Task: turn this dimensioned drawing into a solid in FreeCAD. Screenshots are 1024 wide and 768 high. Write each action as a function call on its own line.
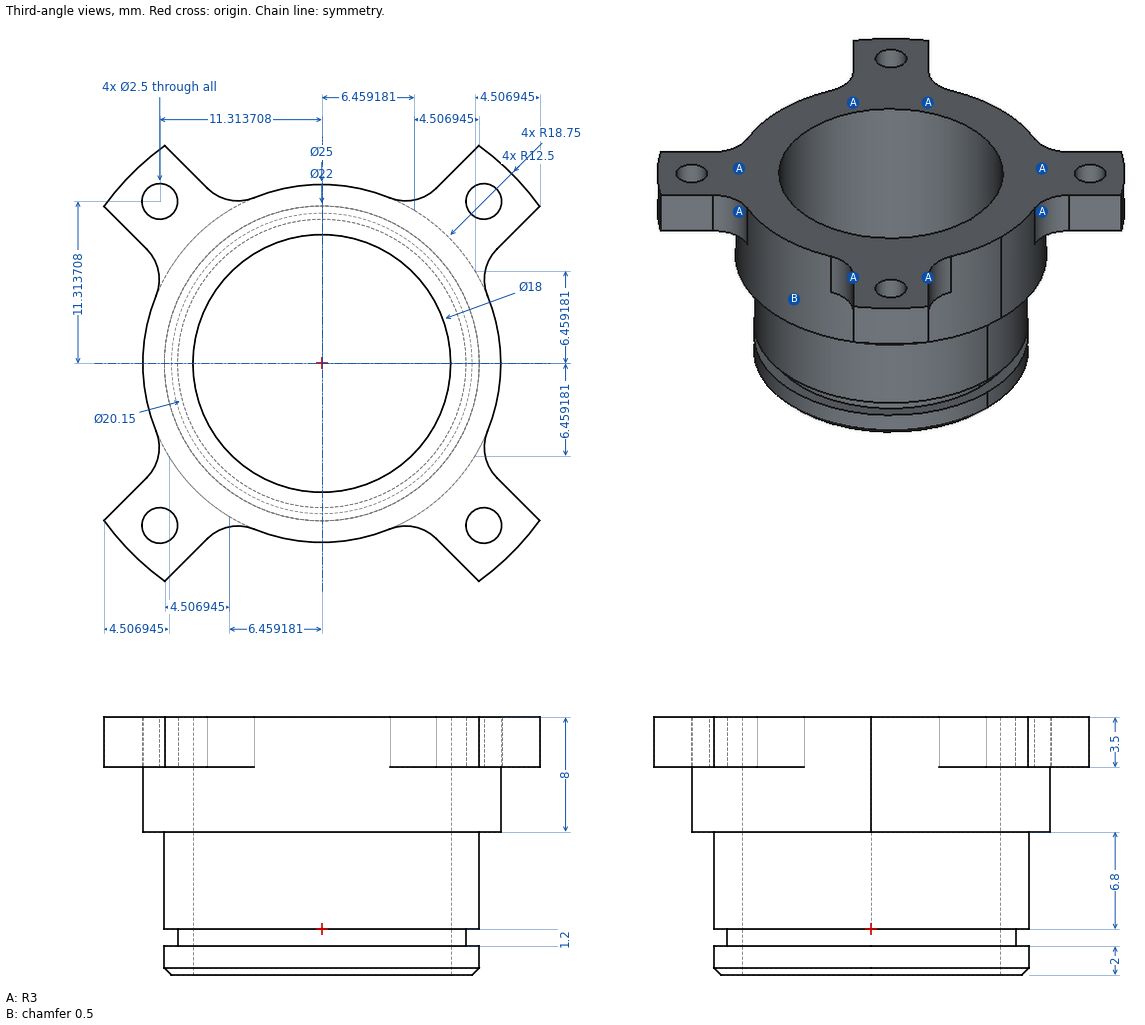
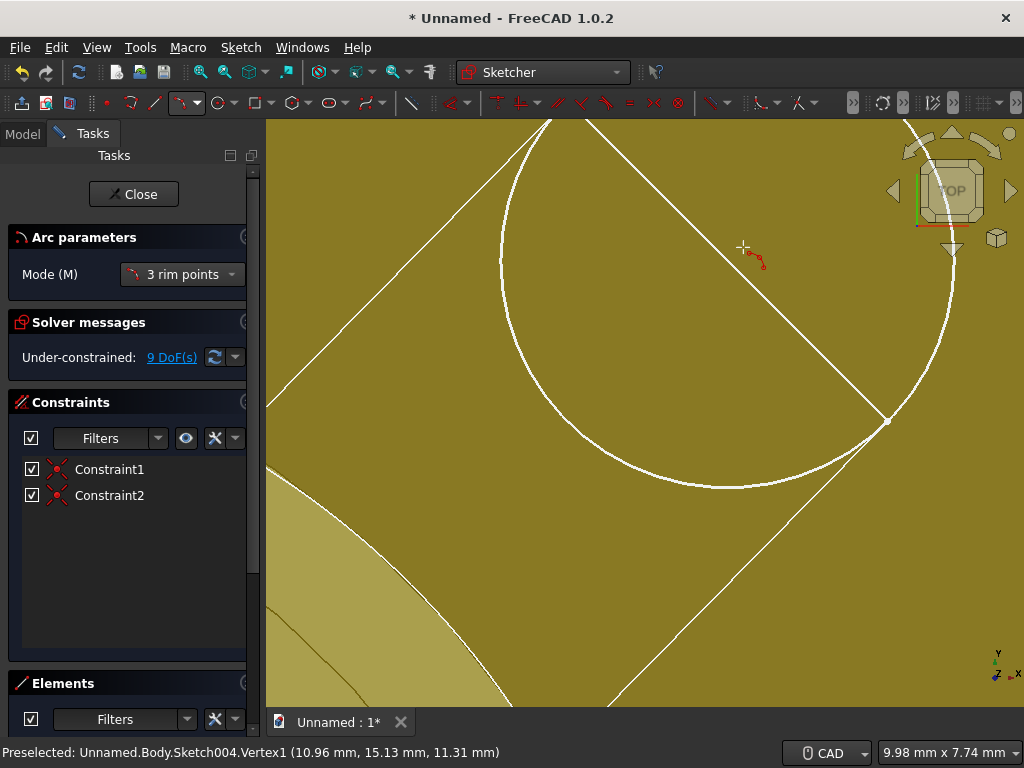
click(742, 243)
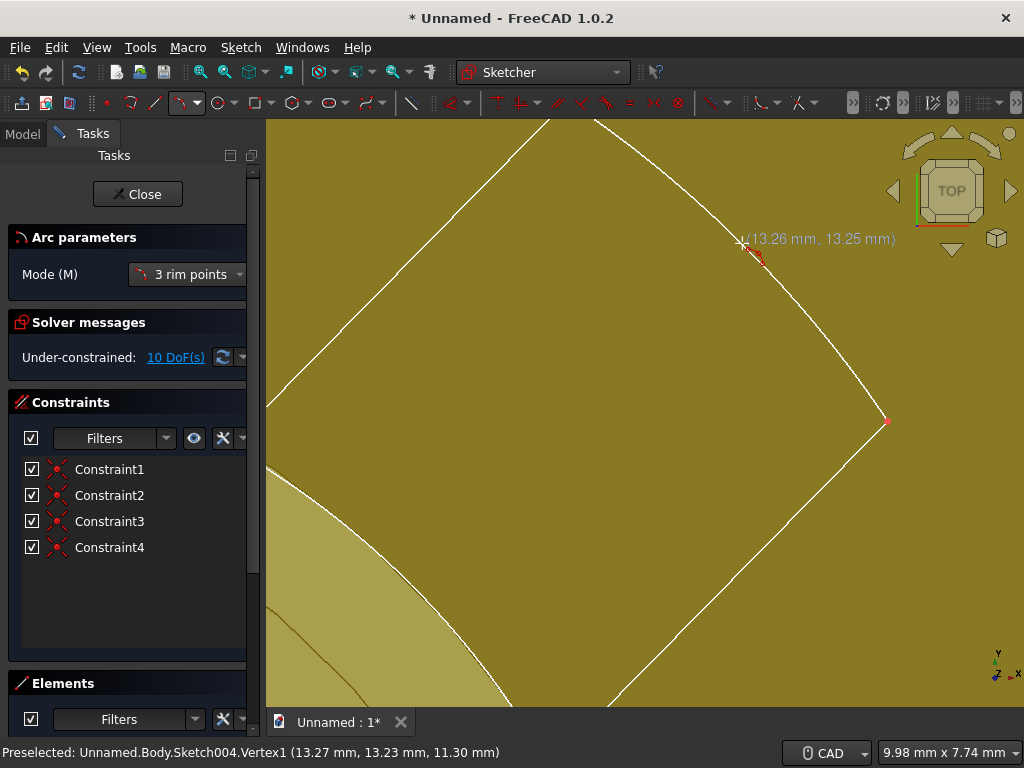
click(156, 104)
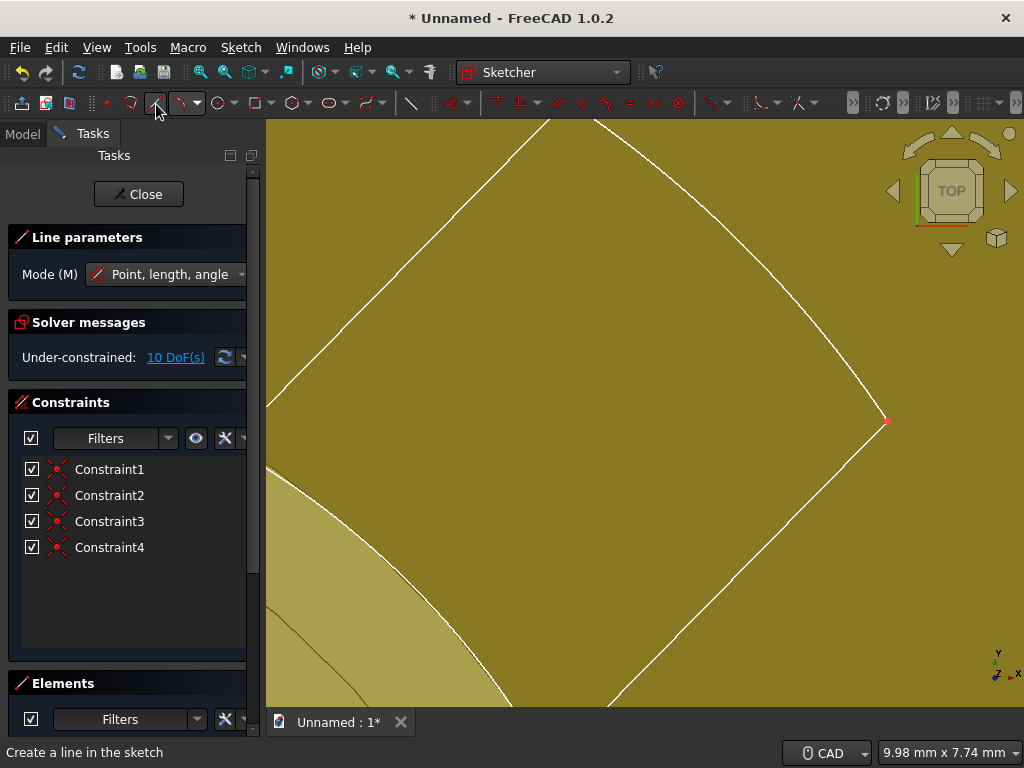
scroll(743, 247, down, 9)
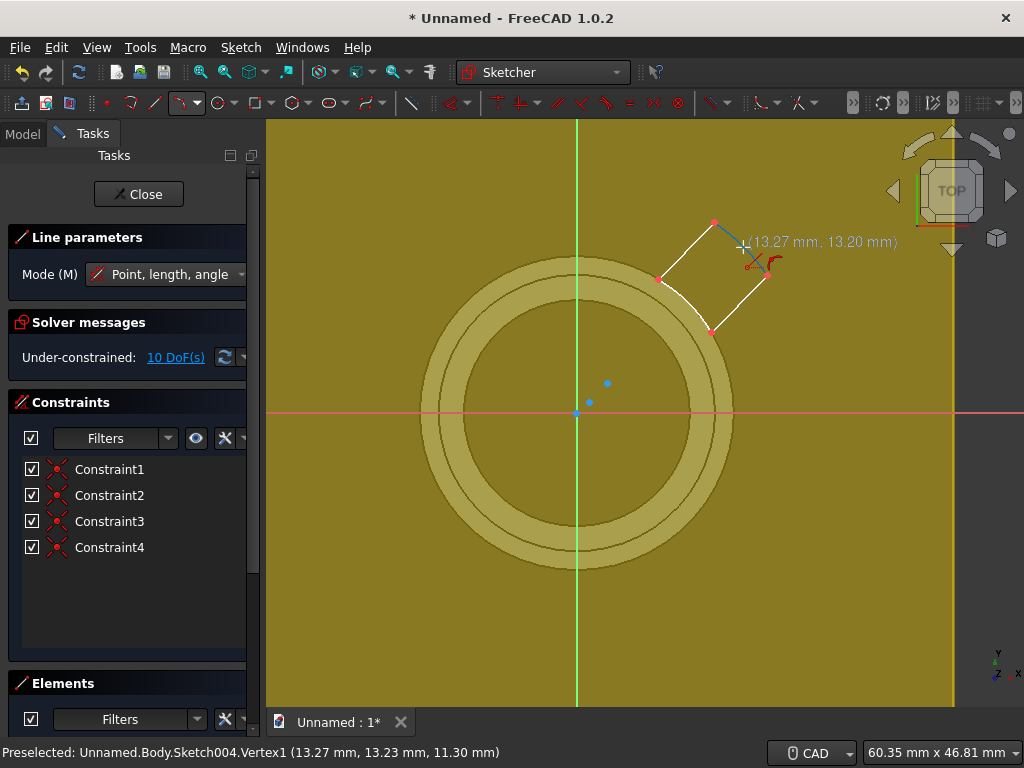
click(768, 551)
click(711, 494)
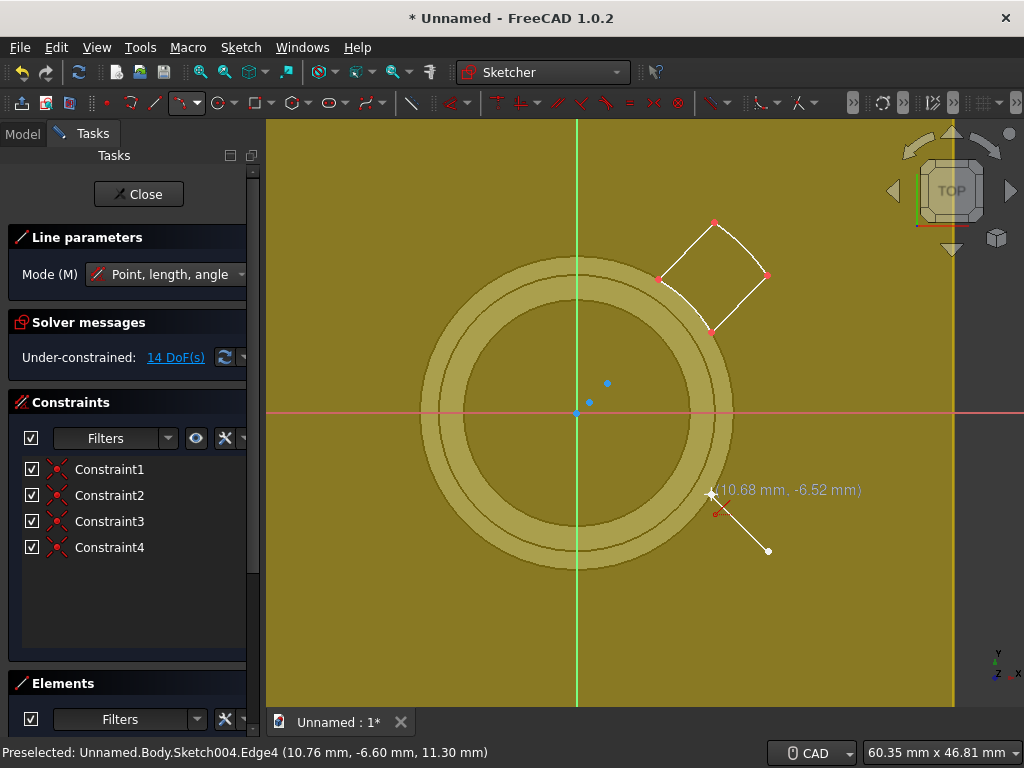
click(658, 548)
click(715, 604)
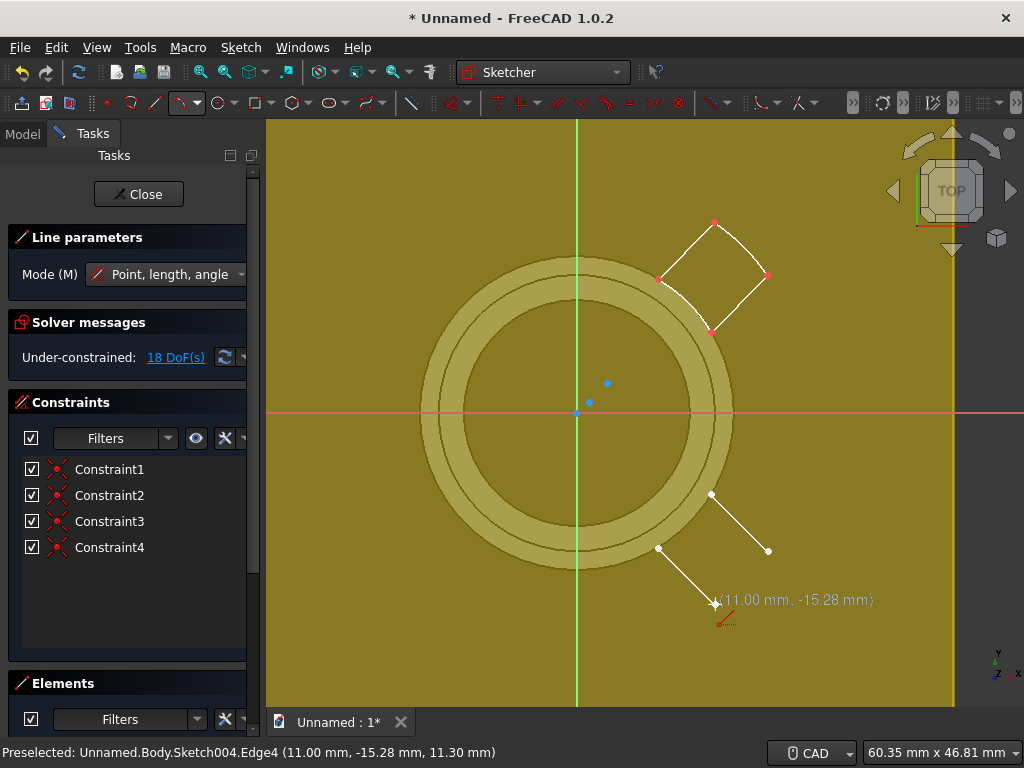
click(180, 104)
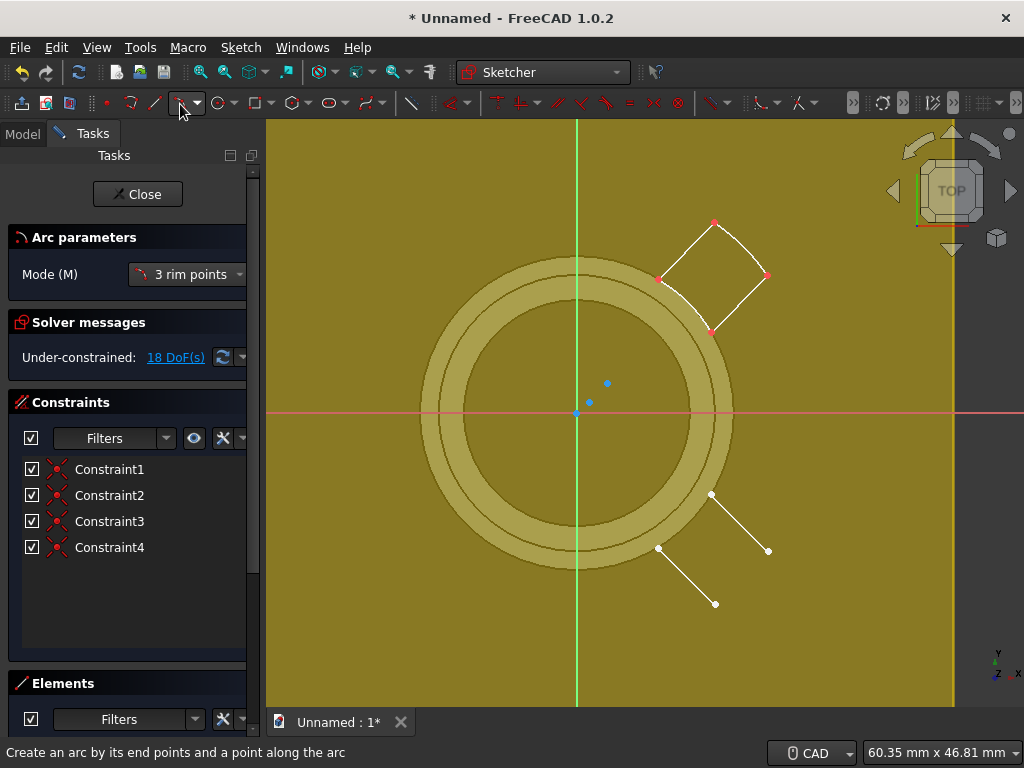
click(711, 495)
click(658, 549)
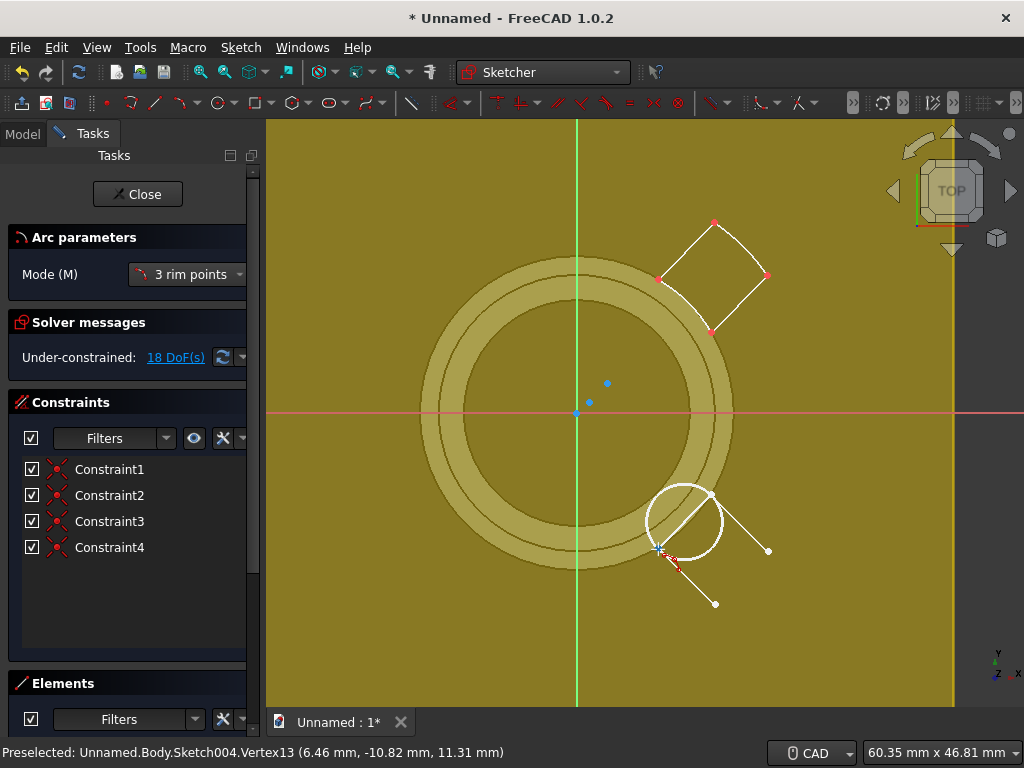
scroll(688, 524, up, 7)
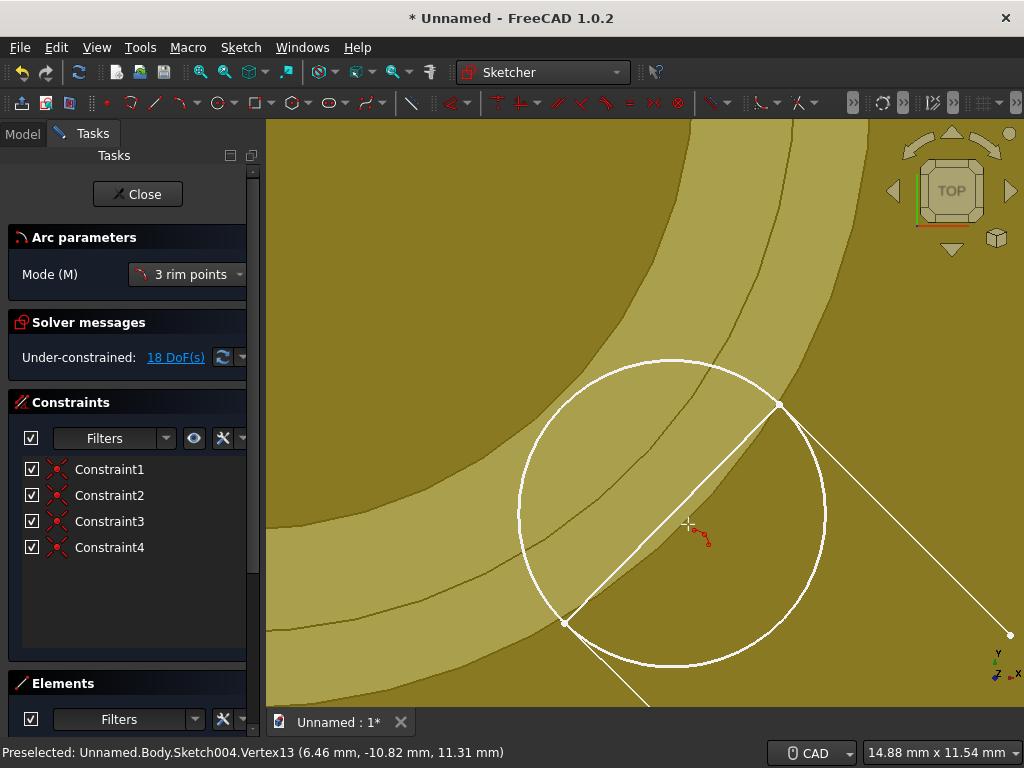
click(686, 522)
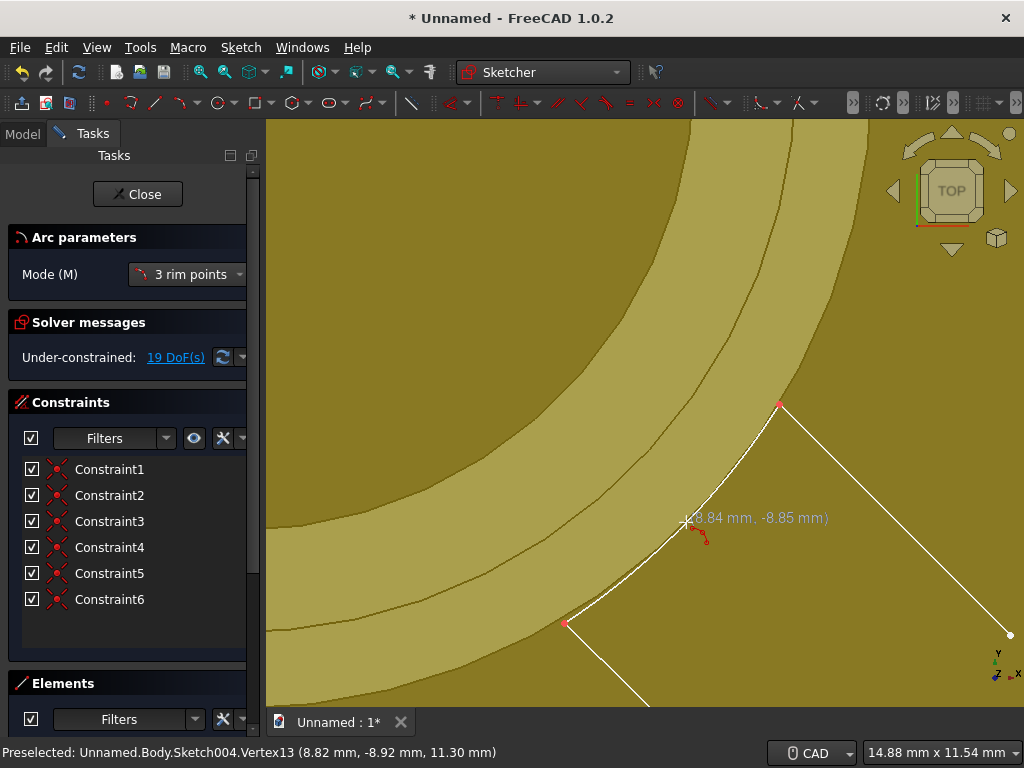
scroll(688, 525, down, 7)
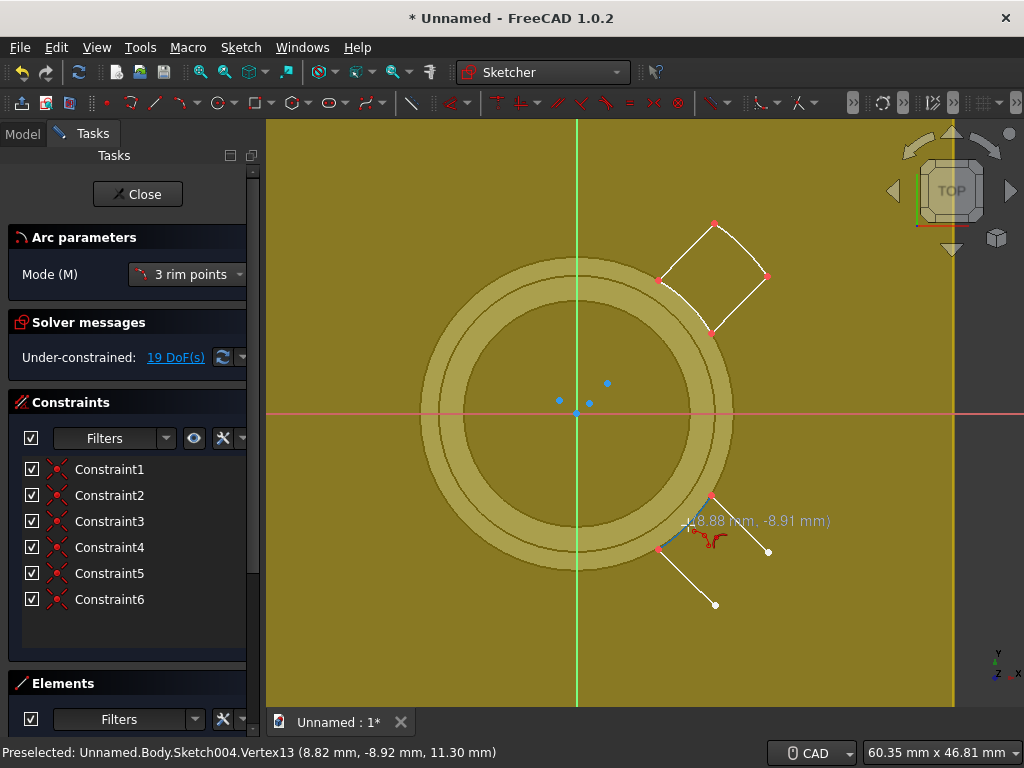
click(715, 606)
click(768, 553)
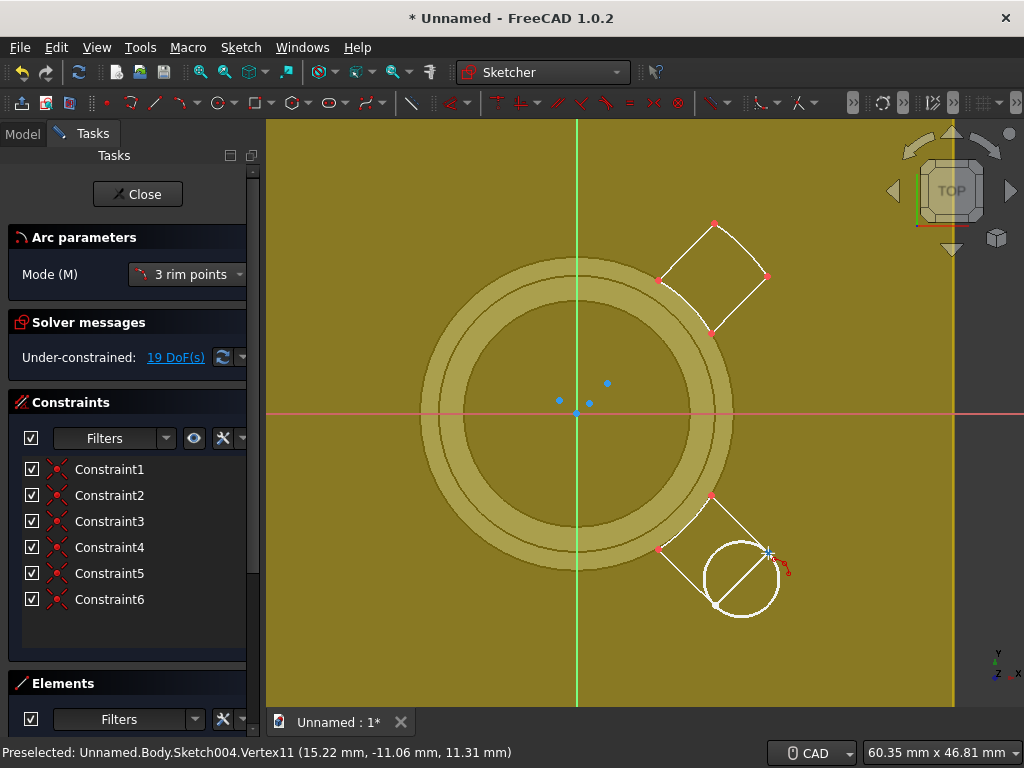
scroll(743, 580, up, 9)